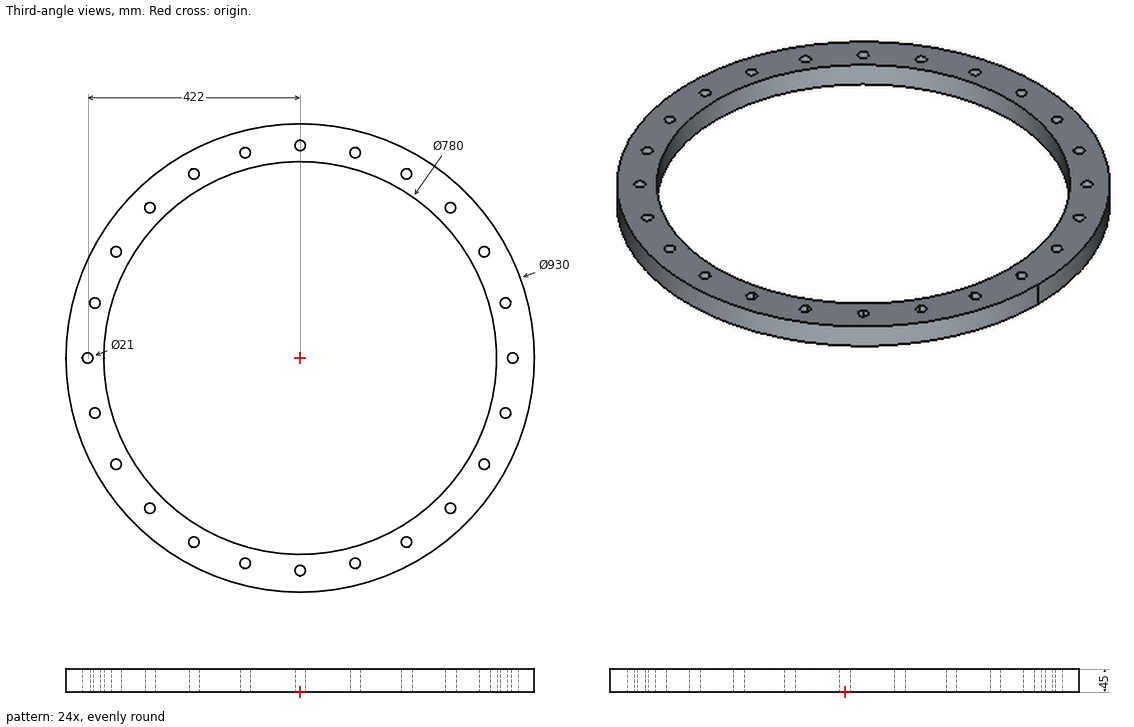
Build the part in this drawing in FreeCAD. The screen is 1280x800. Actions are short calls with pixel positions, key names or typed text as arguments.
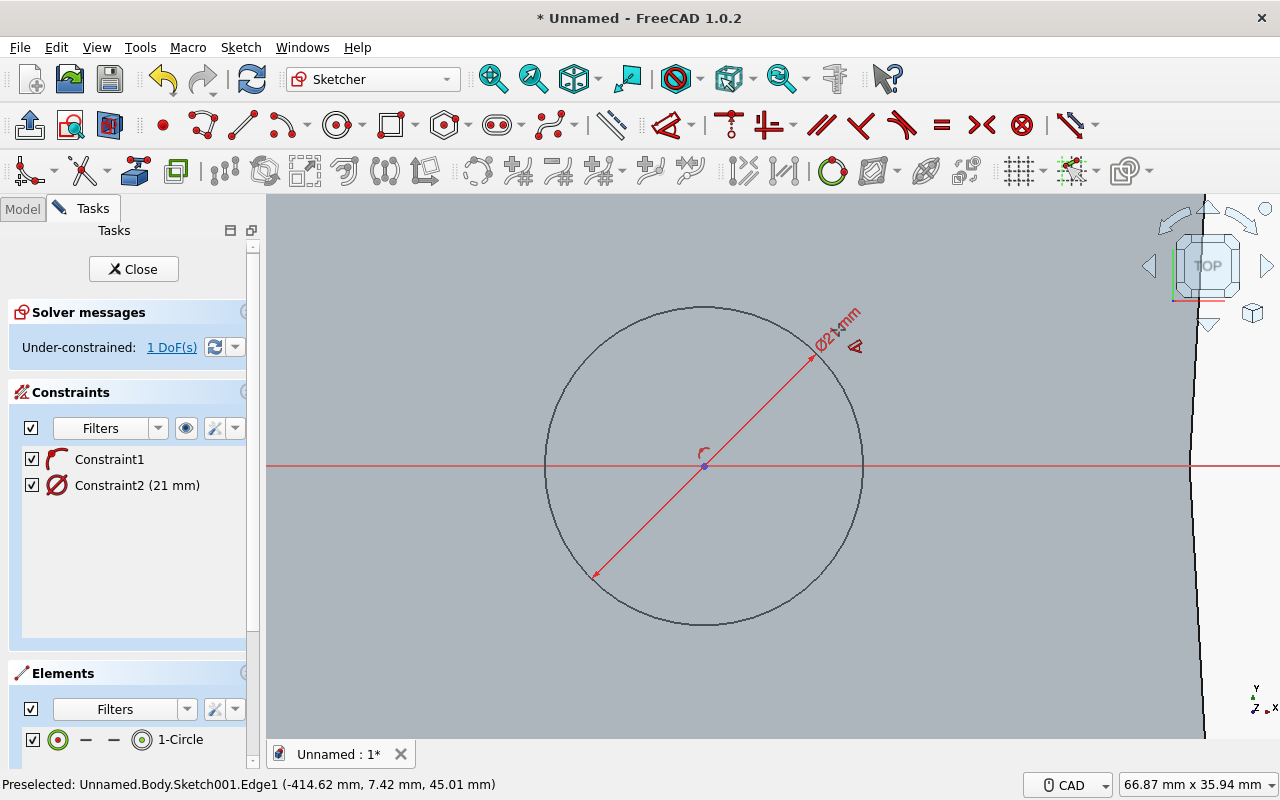
click(704, 466)
click(910, 500)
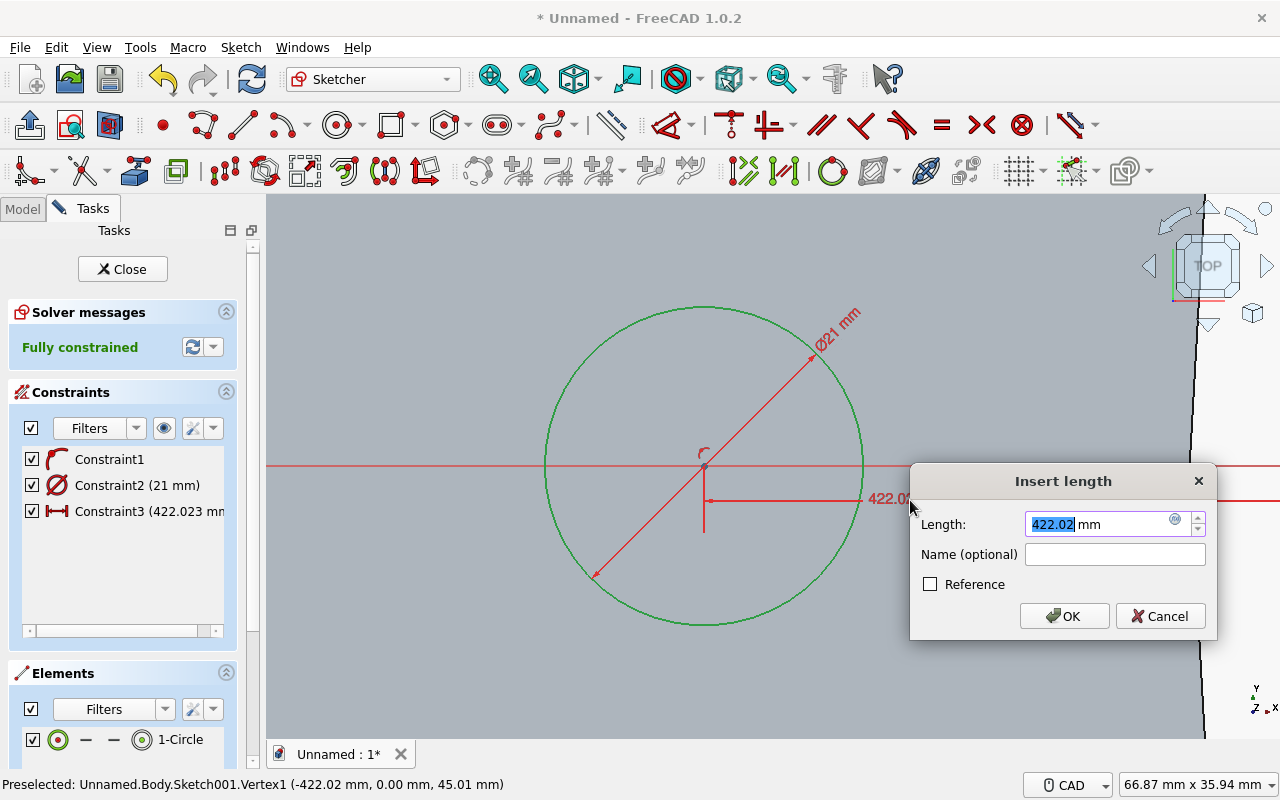
text(422)
key(Return)
key(Escape)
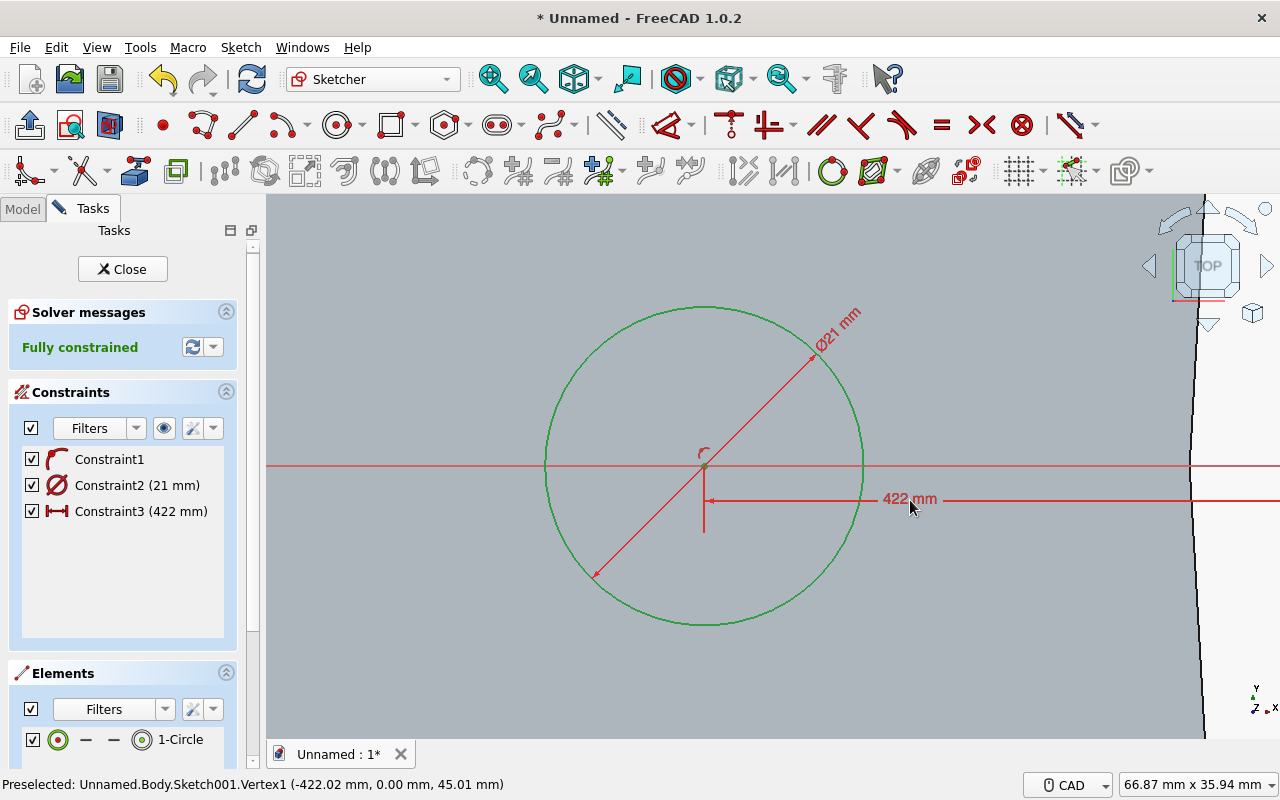
click(123, 269)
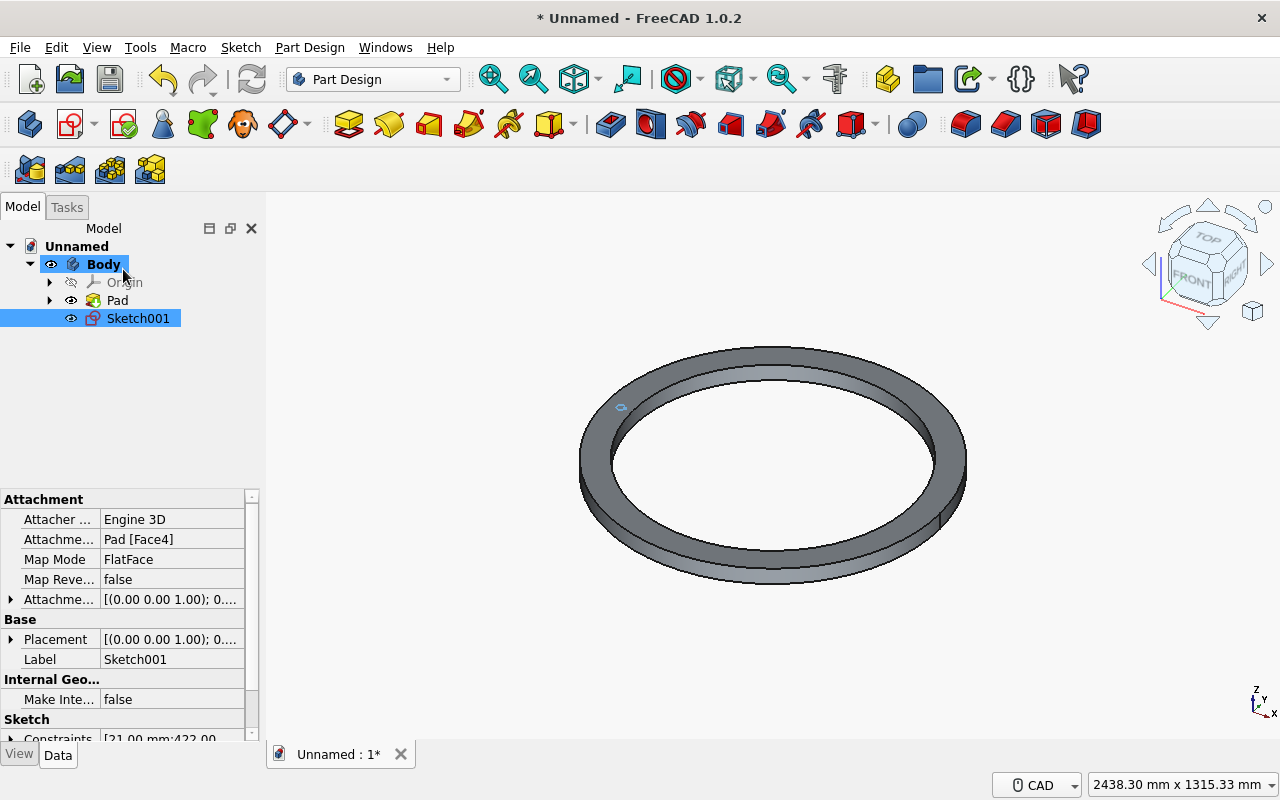
click(612, 124)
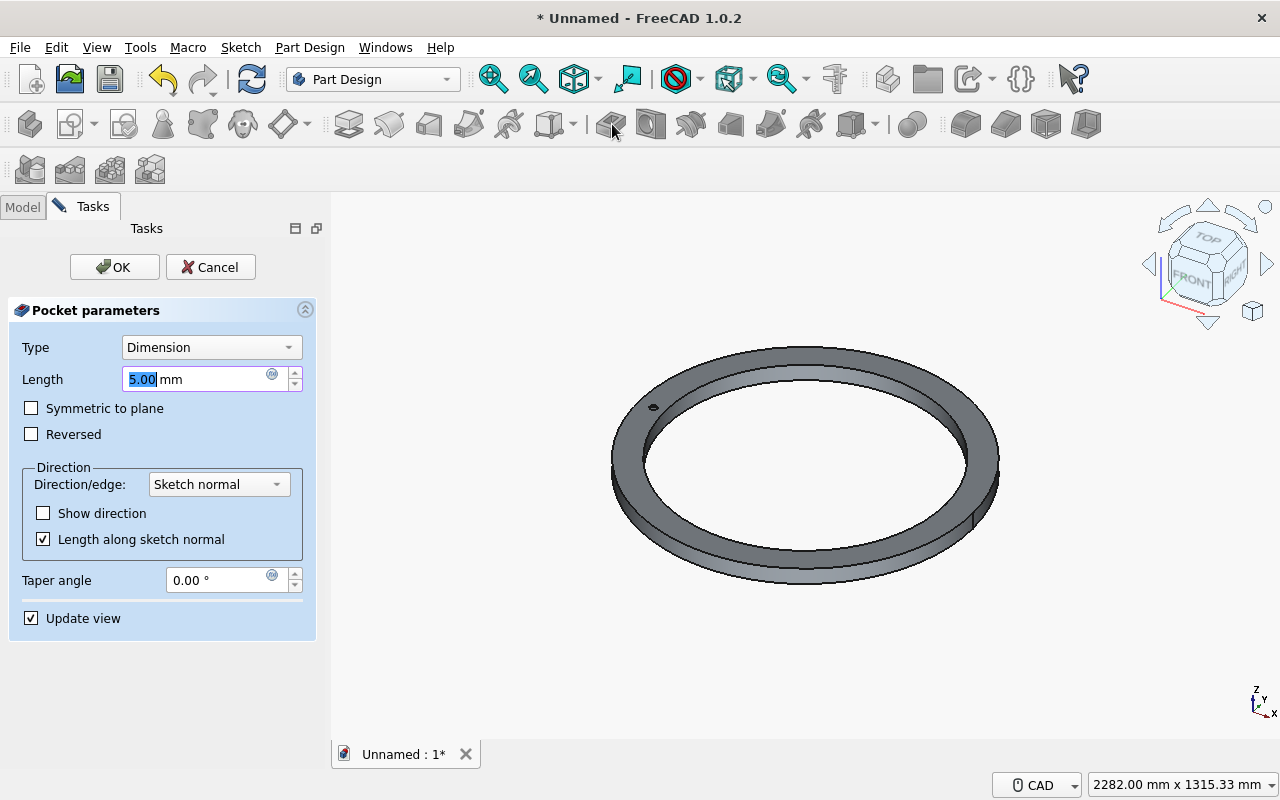
click(212, 348)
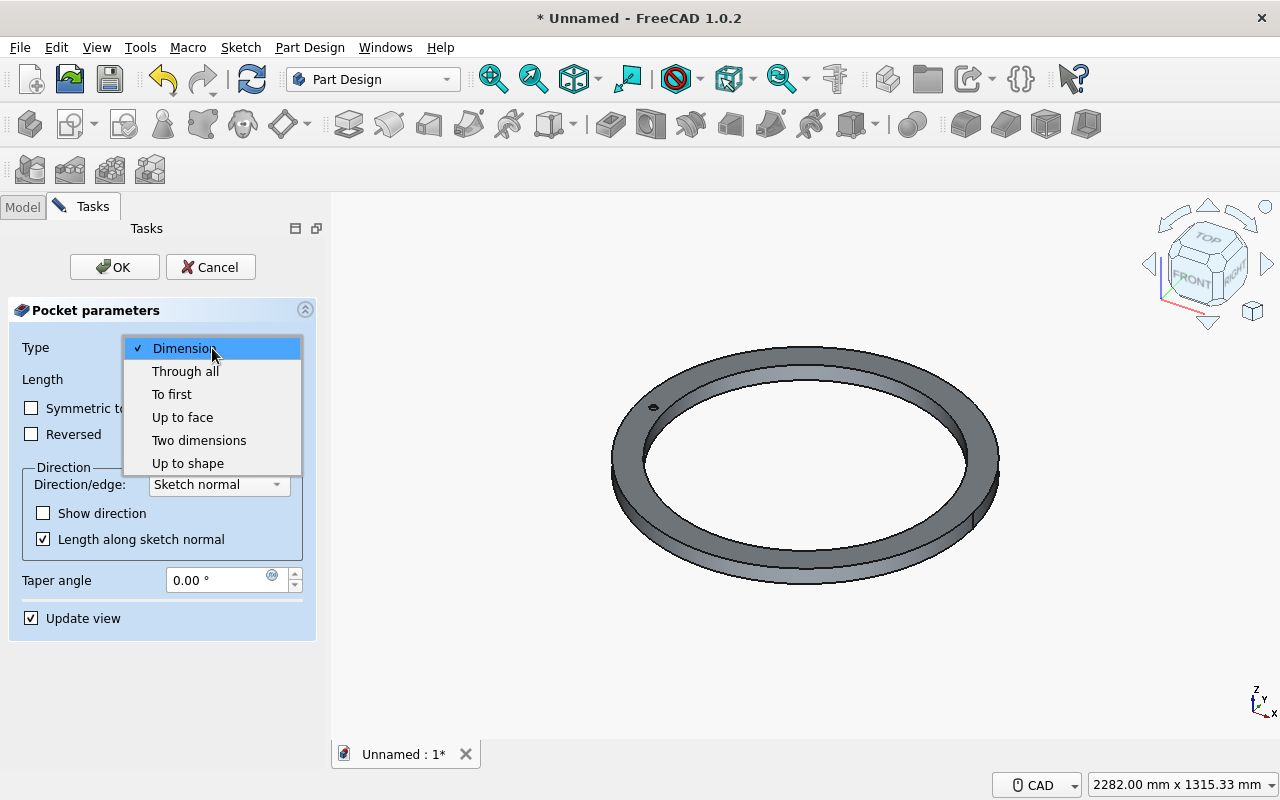
click(212, 372)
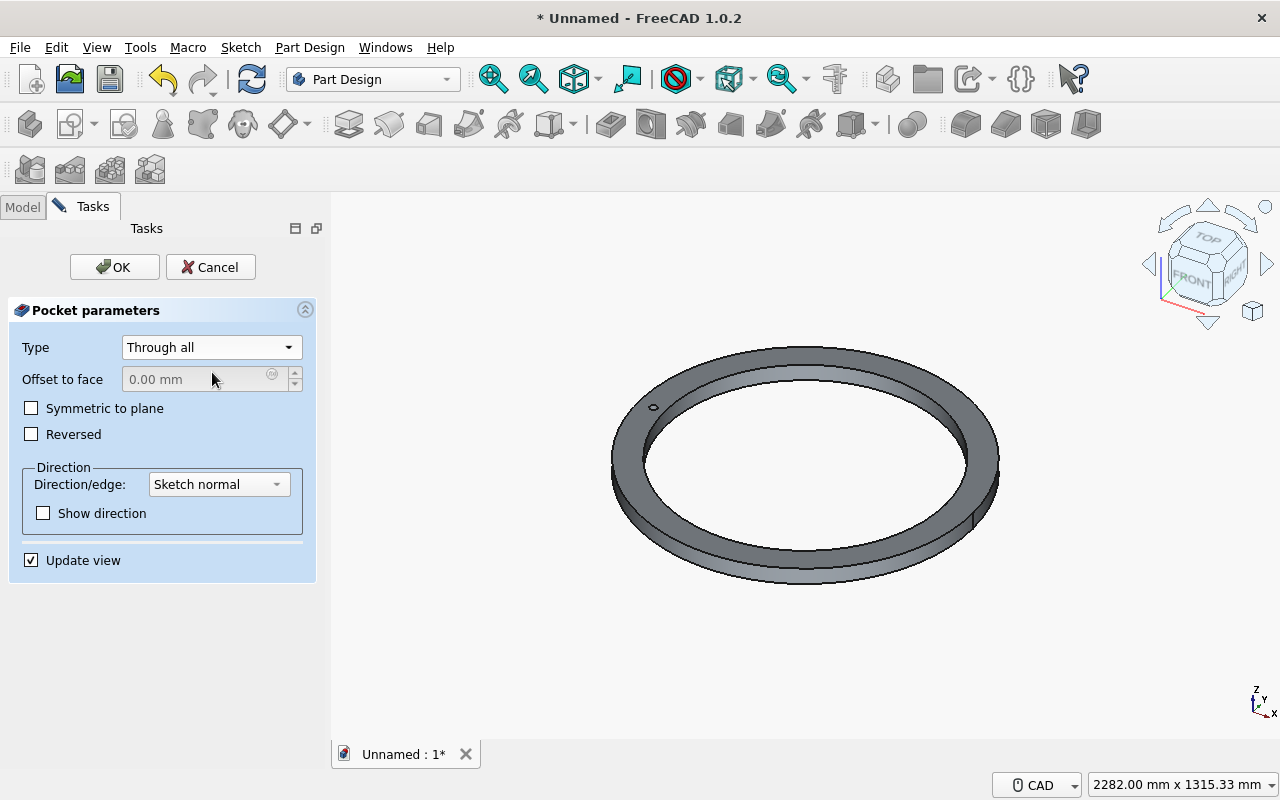
click(115, 267)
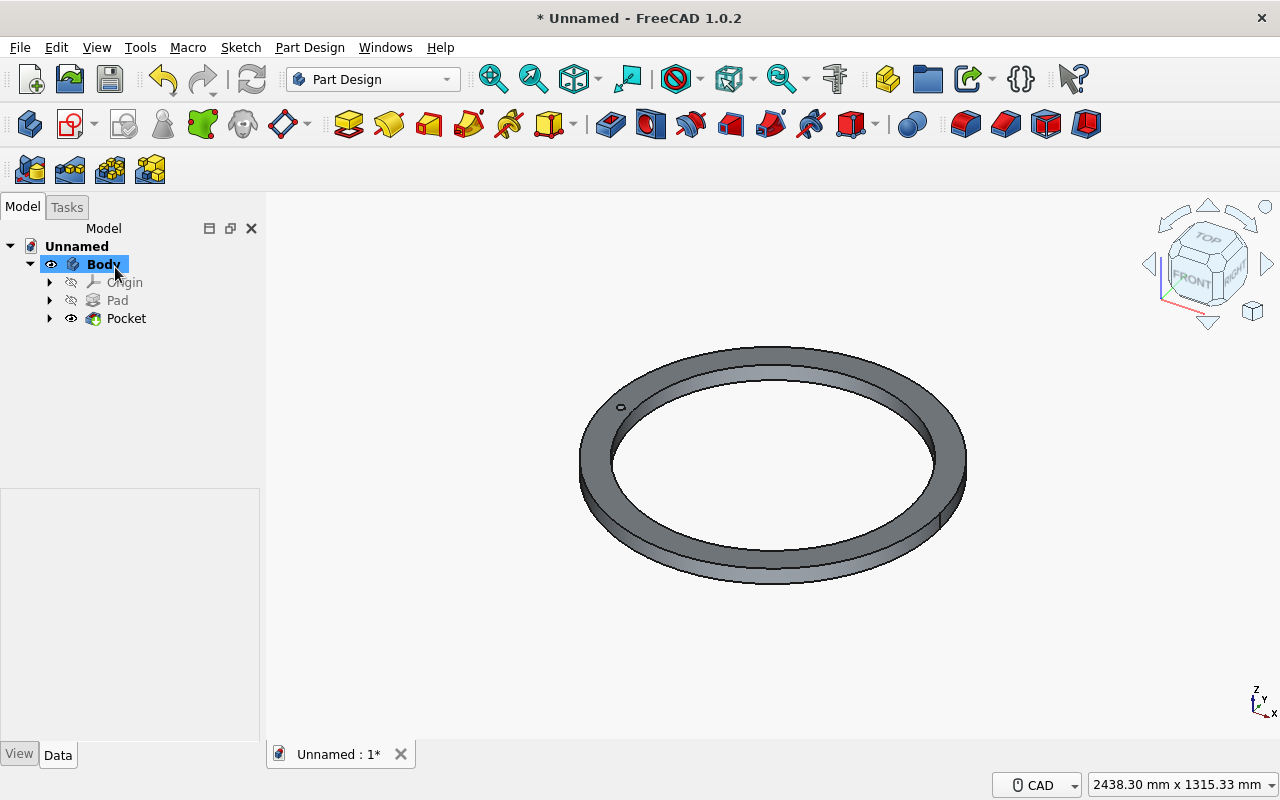
click(116, 318)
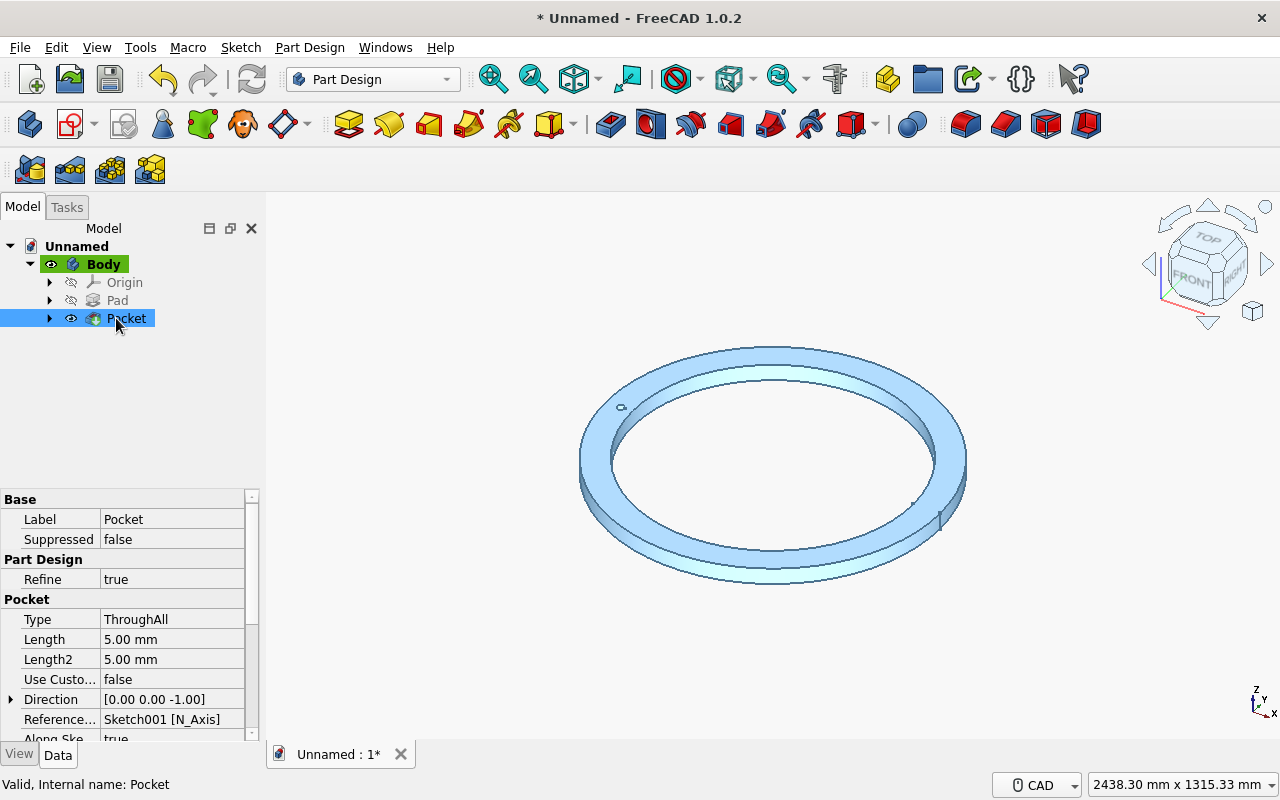
click(110, 170)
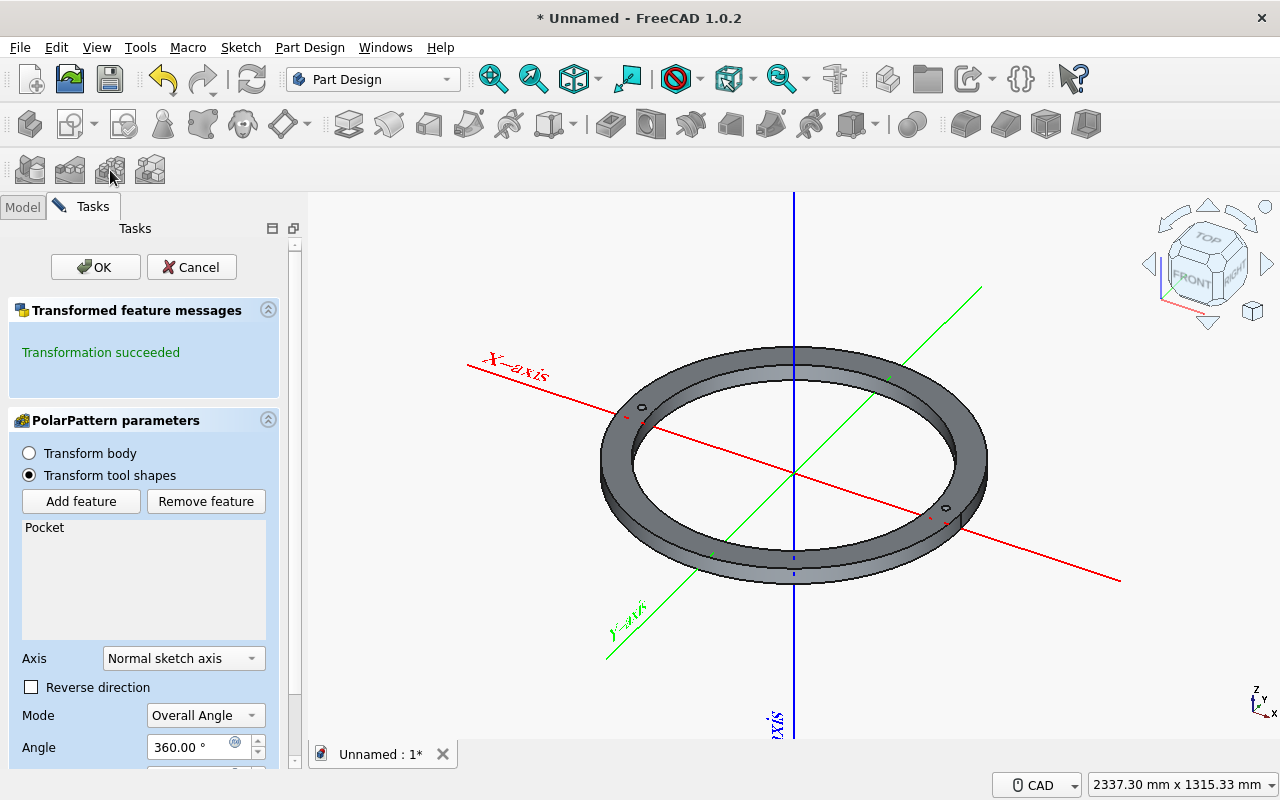
click(184, 658)